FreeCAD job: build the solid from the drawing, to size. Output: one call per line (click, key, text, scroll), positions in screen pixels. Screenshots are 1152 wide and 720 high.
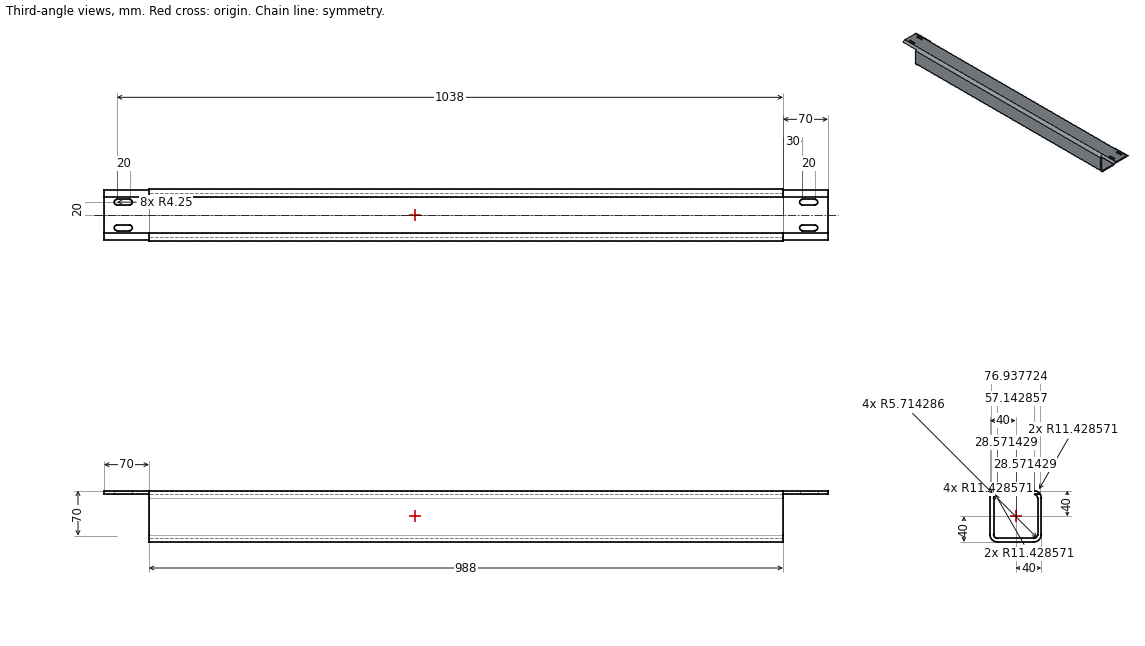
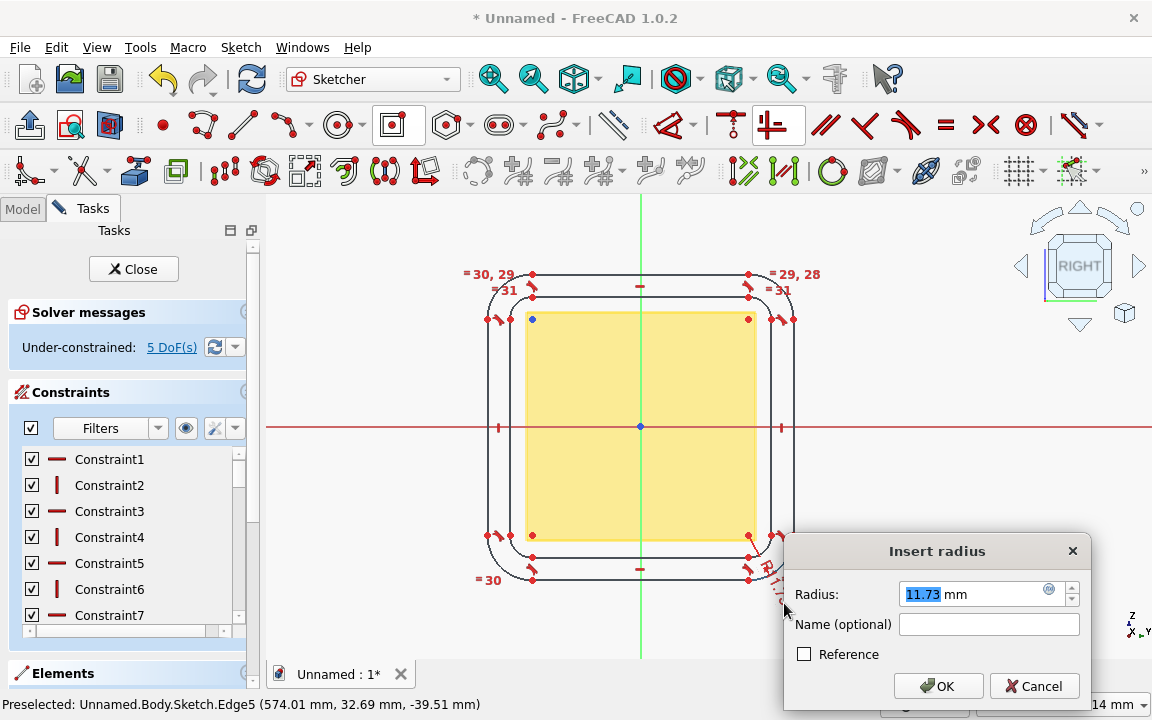
text(11.428571)
key(Return)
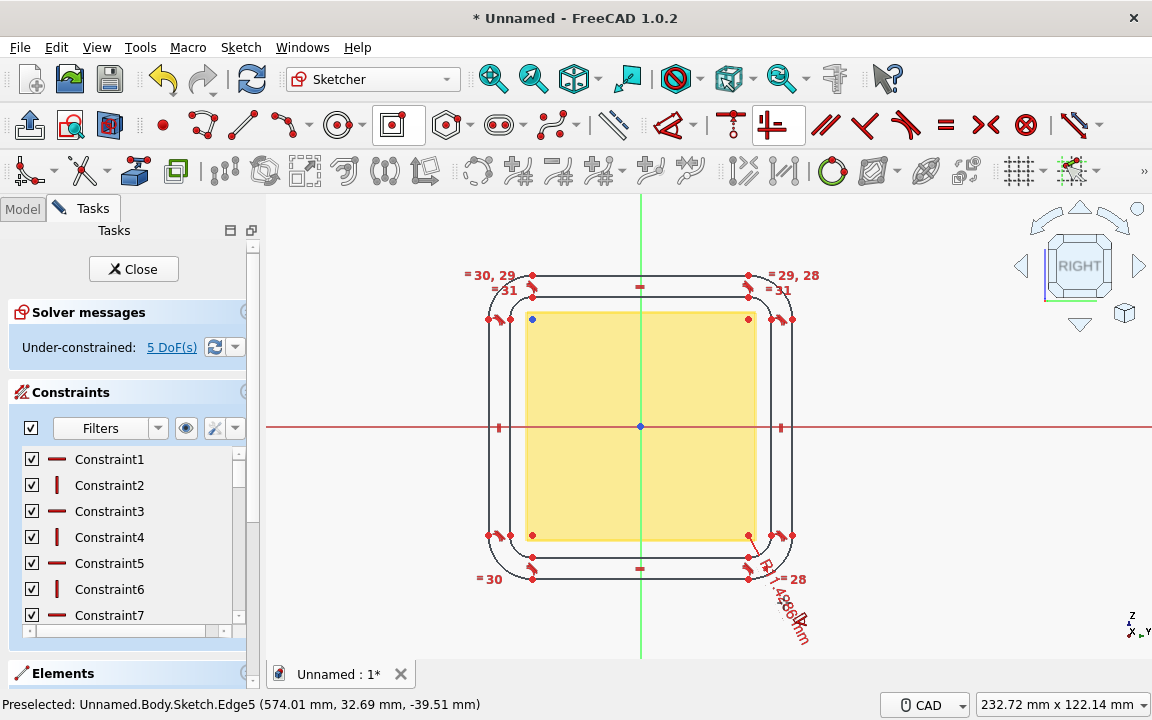
scroll(769, 309, up, 4)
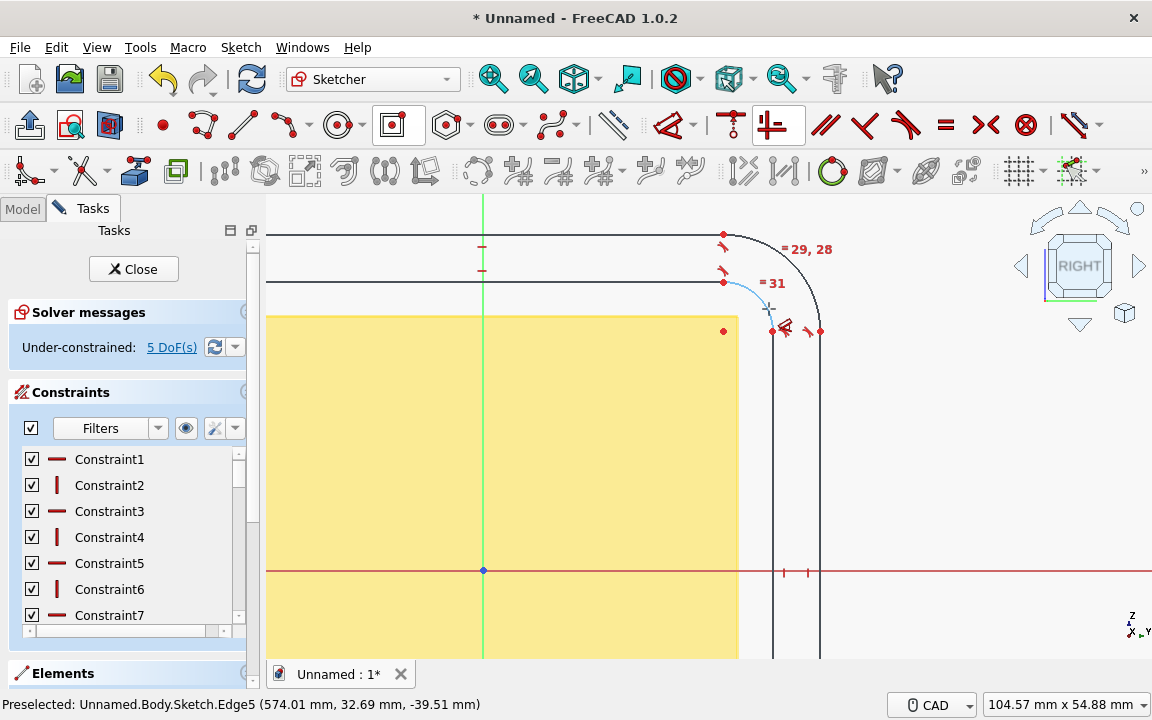
click(768, 309)
click(797, 295)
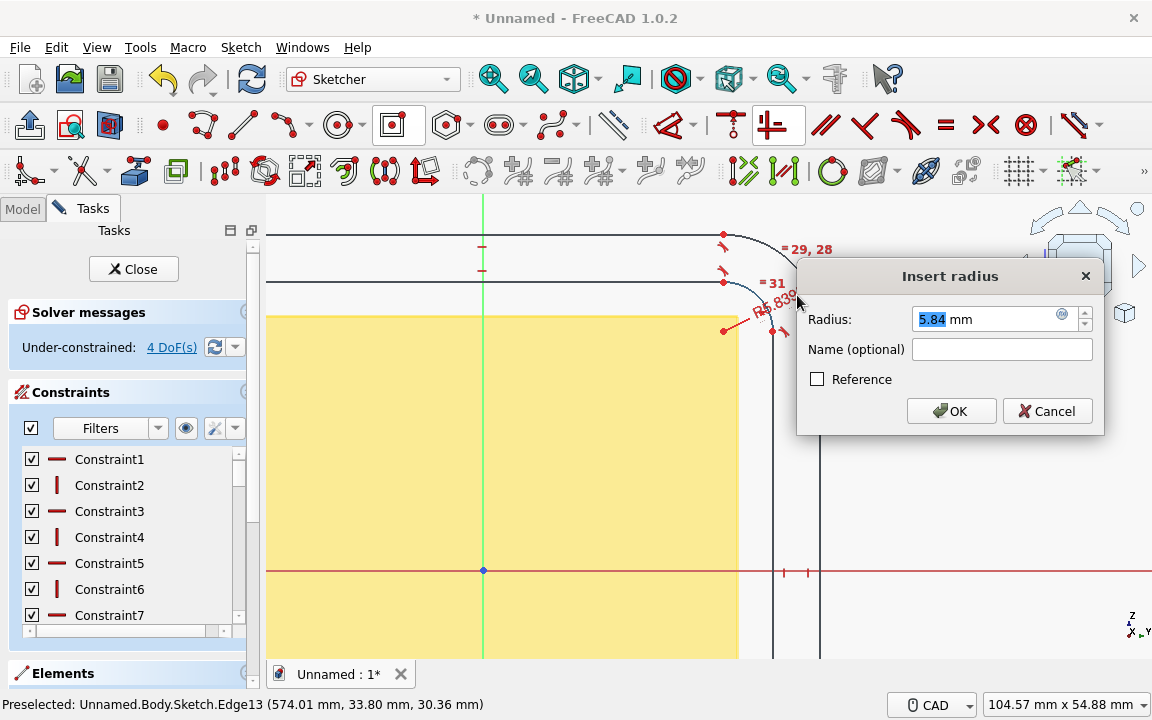
text(5.714286)
key(Return)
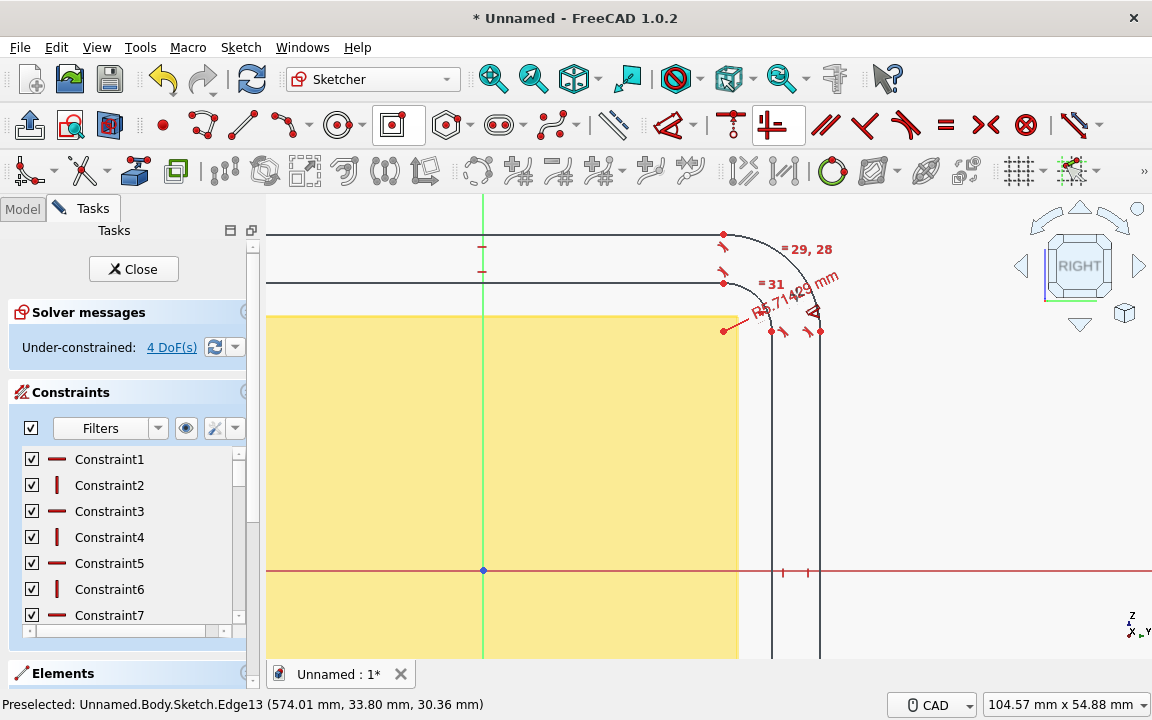
scroll(769, 309, down, 4)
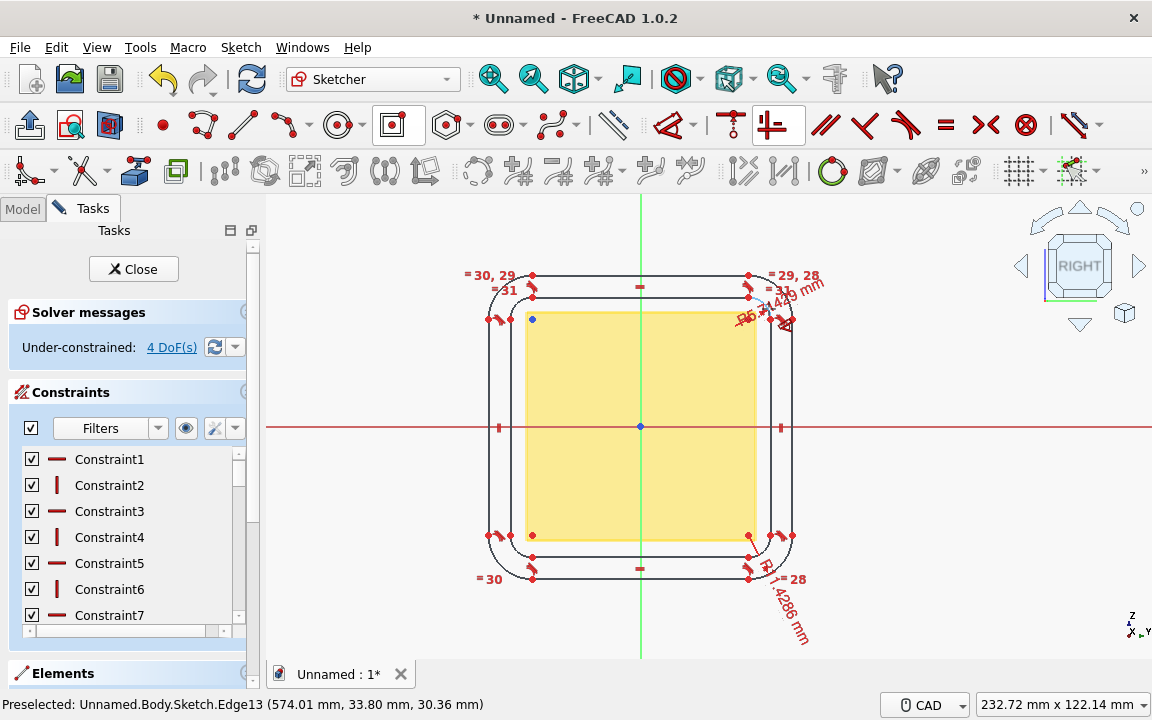
click(532, 579)
click(675, 503)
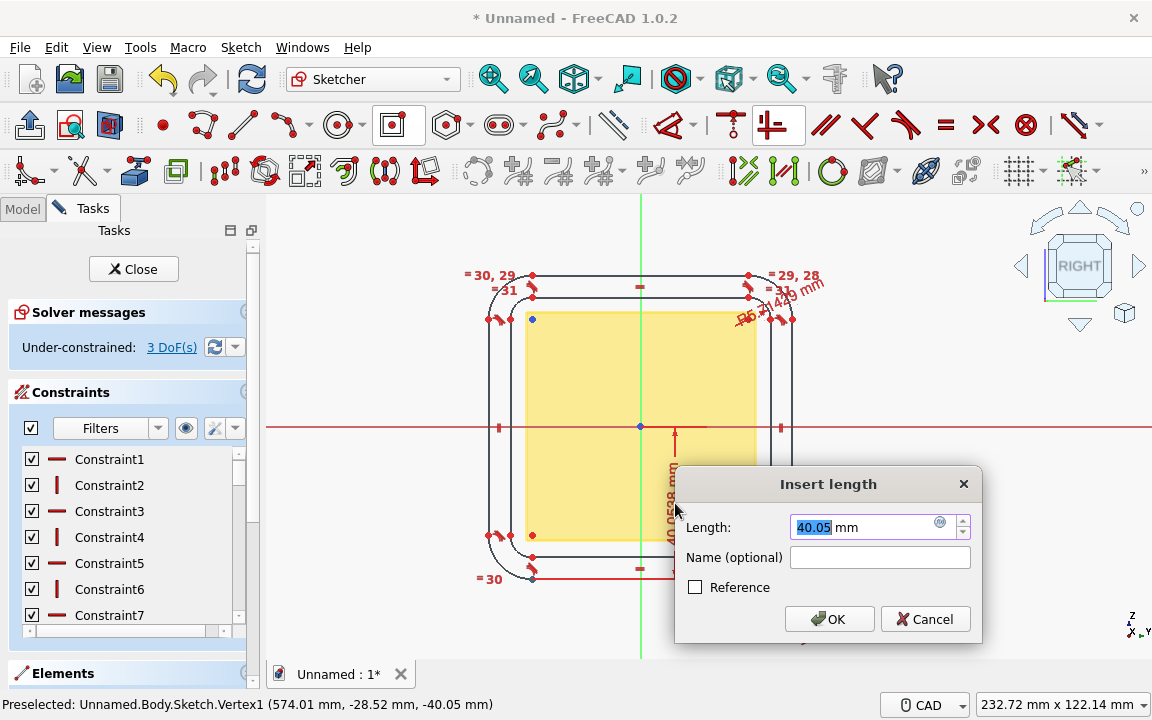
text(40)
key(Return)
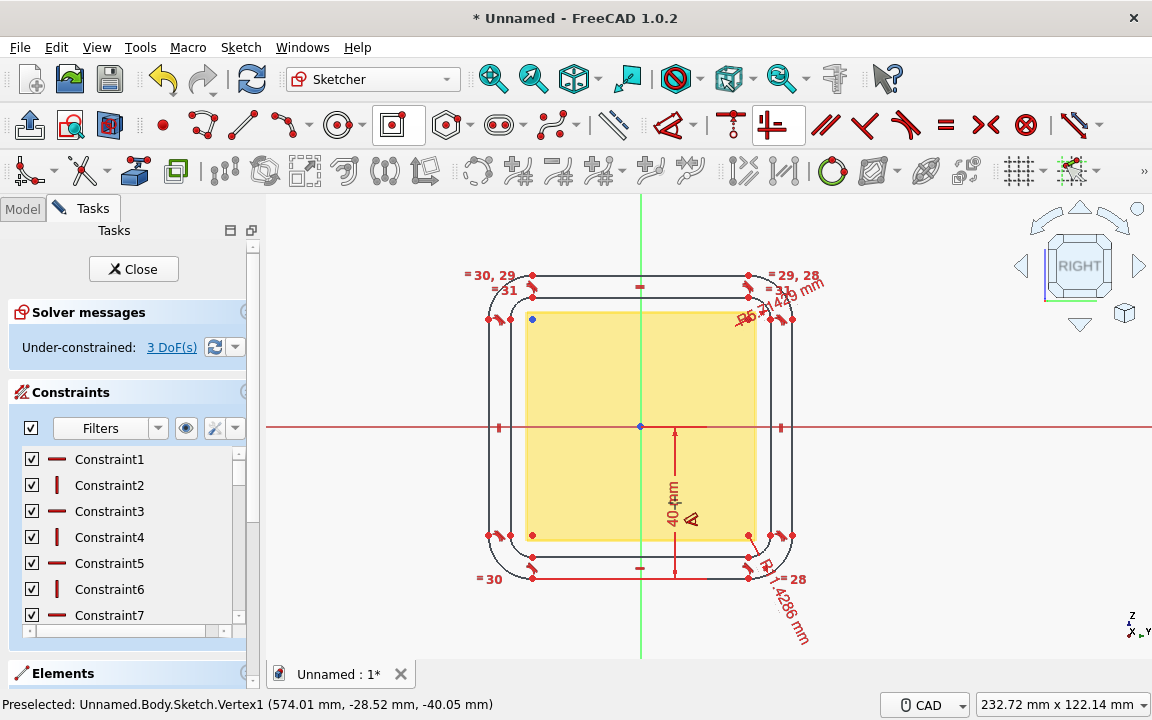
click(792, 535)
click(717, 393)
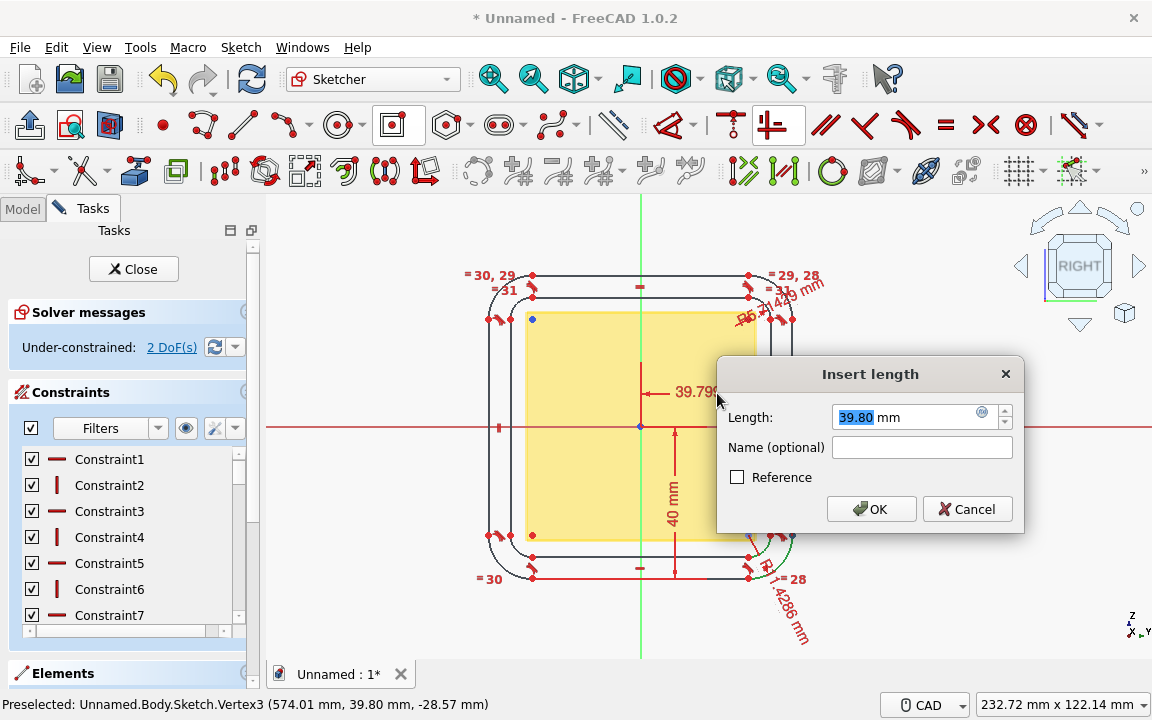
text(40)
key(Return)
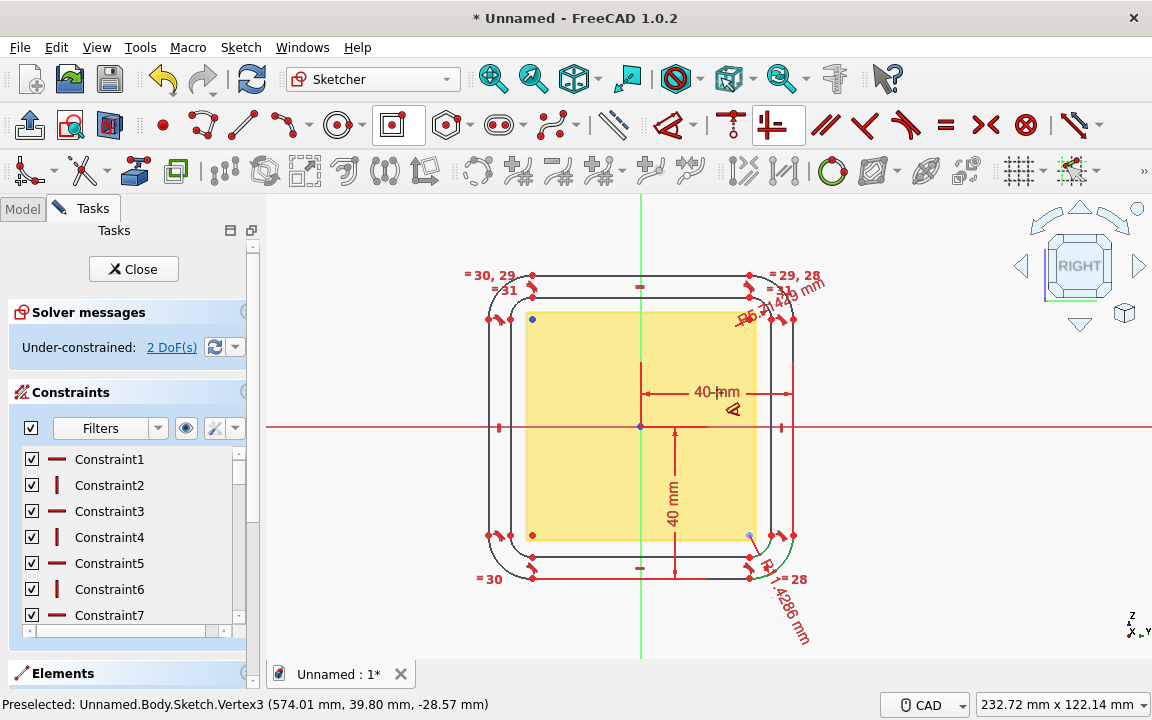
click(750, 276)
click(607, 351)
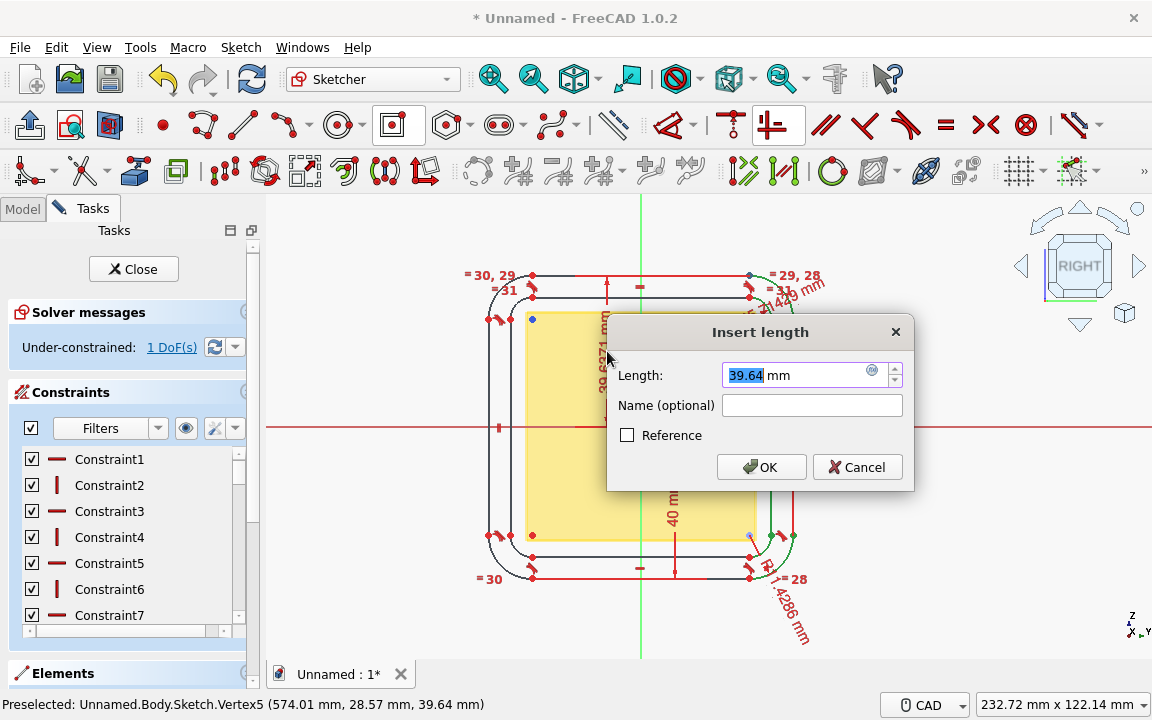
text(40)
key(Return)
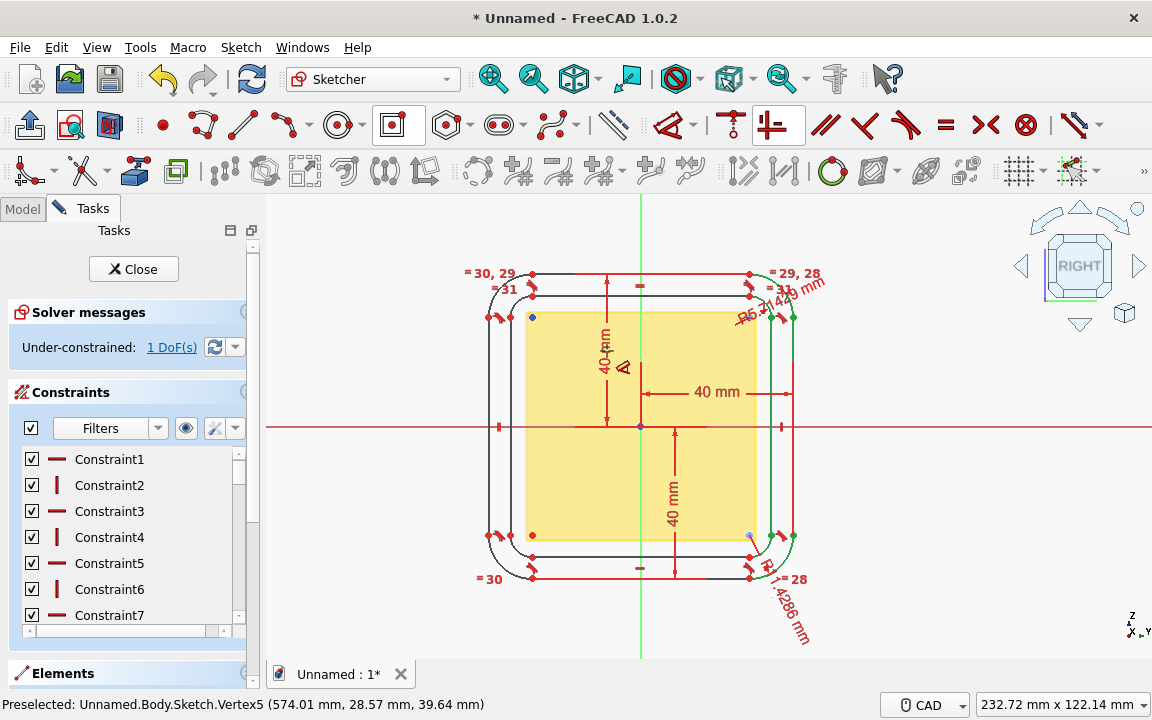
click(489, 318)
click(565, 461)